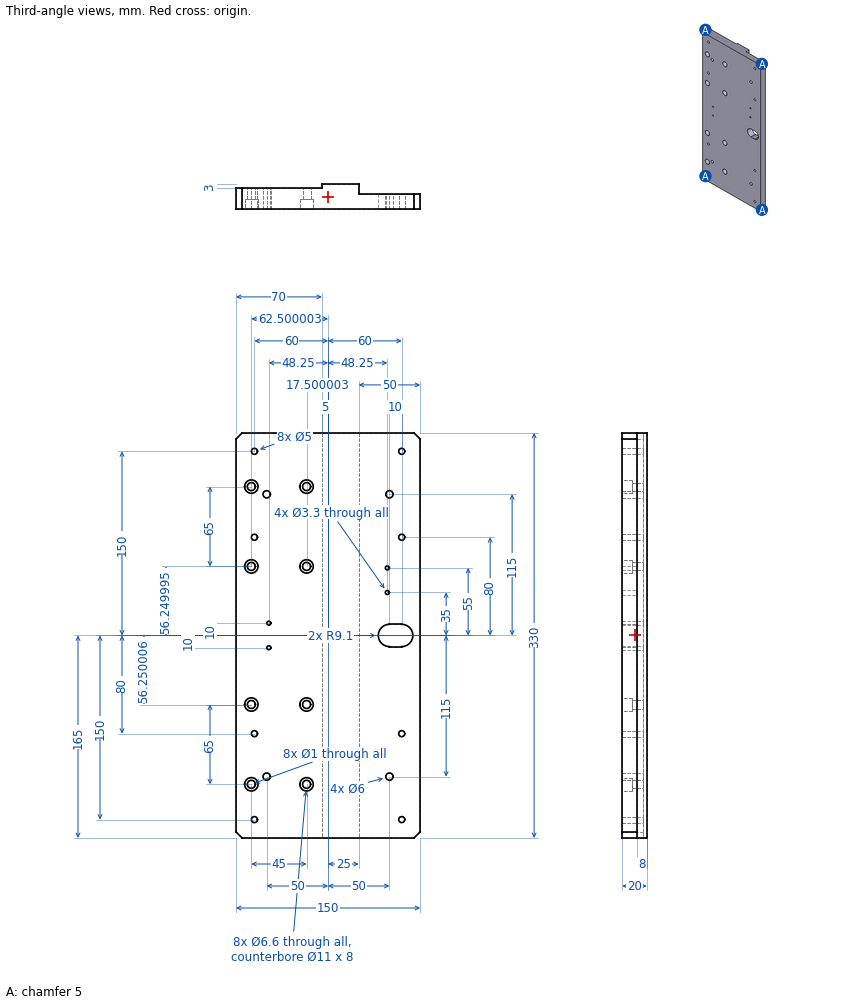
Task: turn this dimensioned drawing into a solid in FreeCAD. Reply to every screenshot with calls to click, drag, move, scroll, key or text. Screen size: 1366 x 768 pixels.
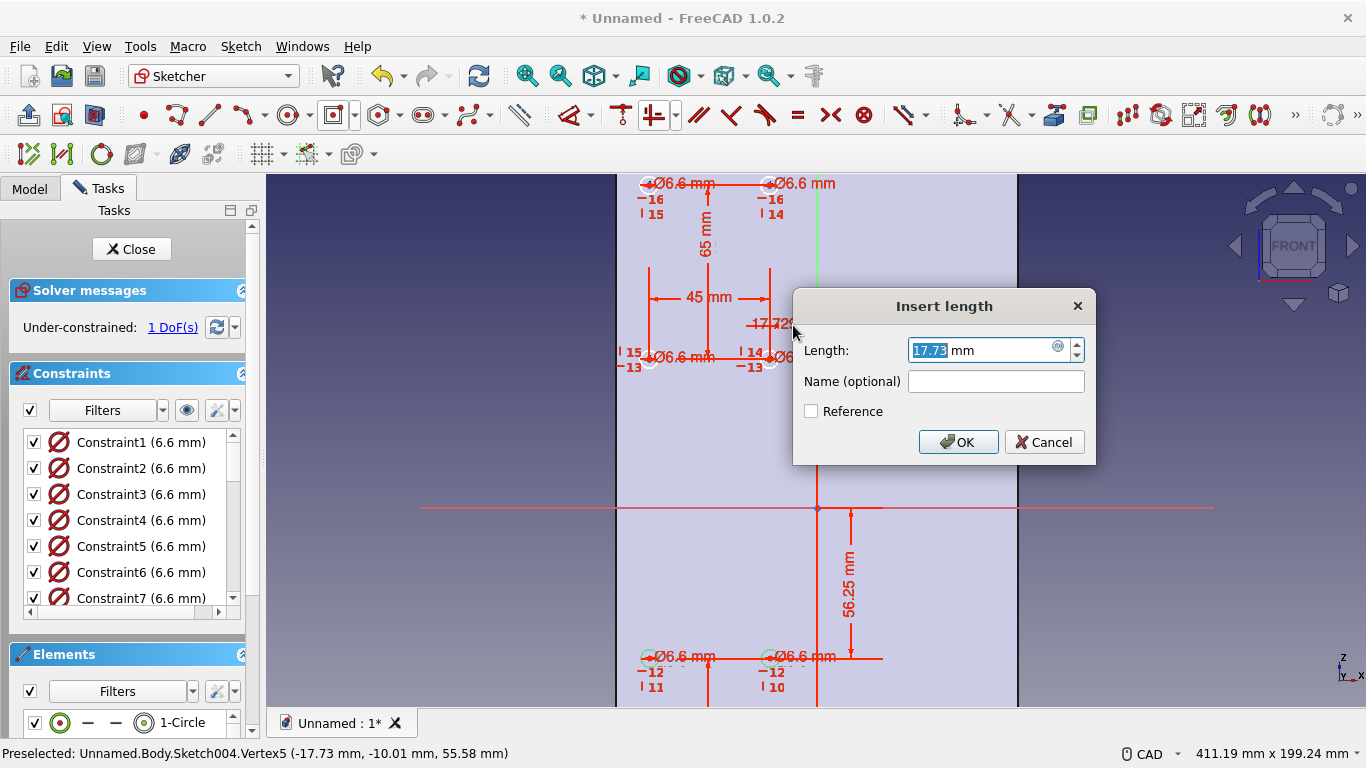
text(17.500003)
key(Return)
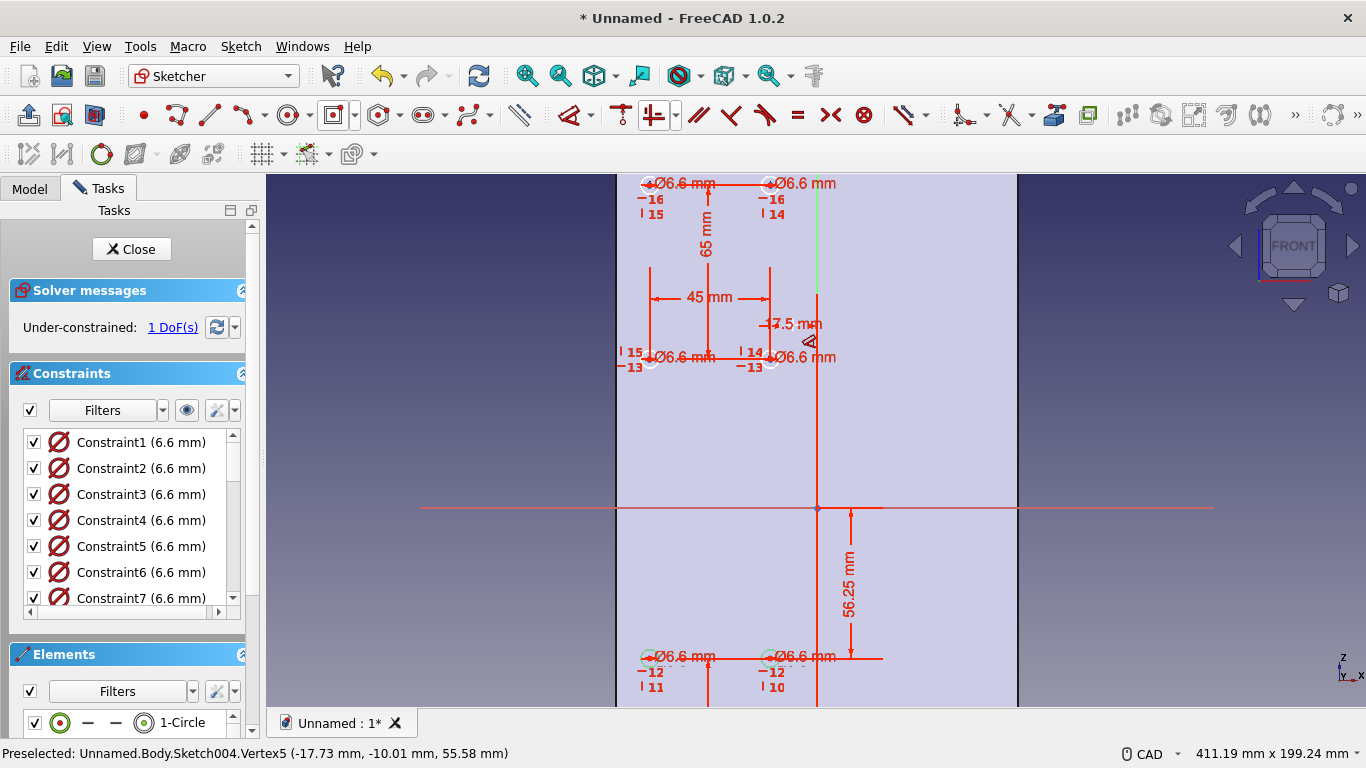
click(770, 359)
click(851, 434)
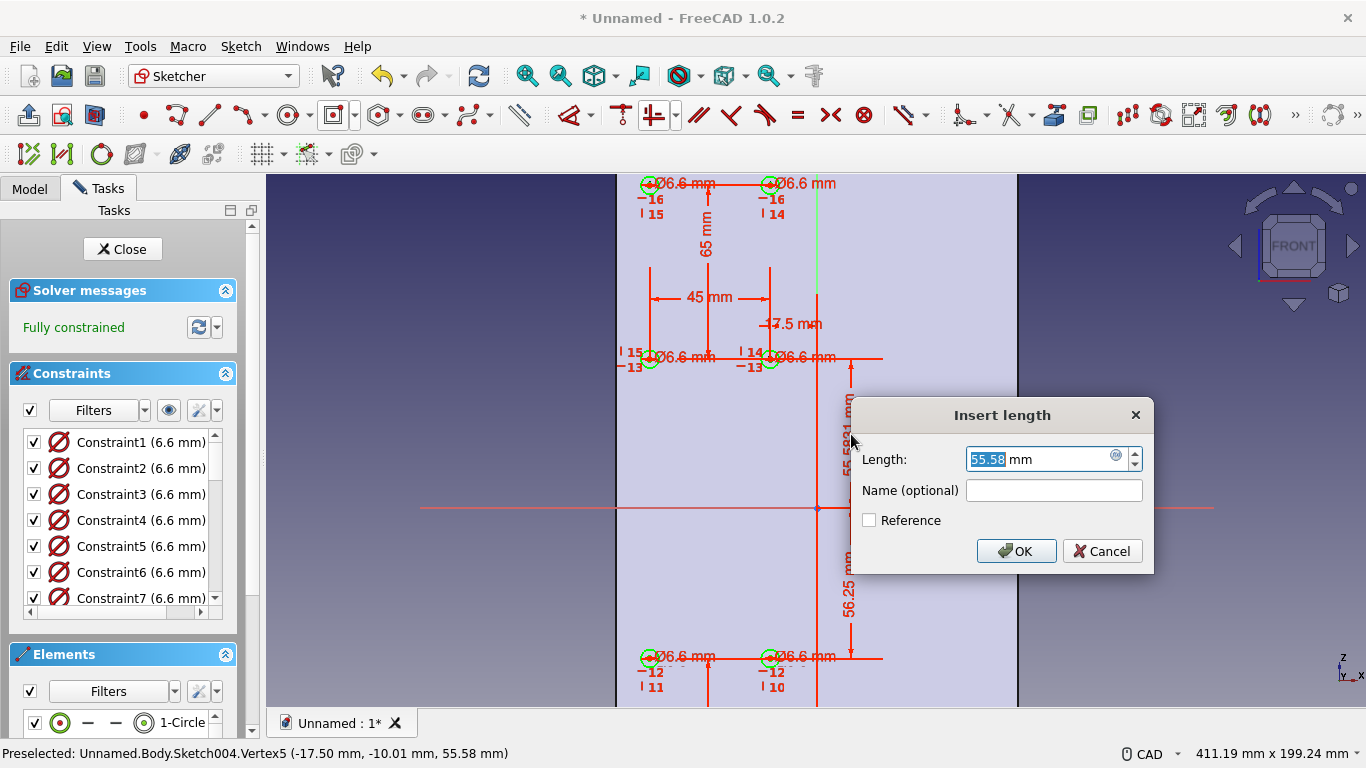
text(56.249995)
key(Return)
key(Escape)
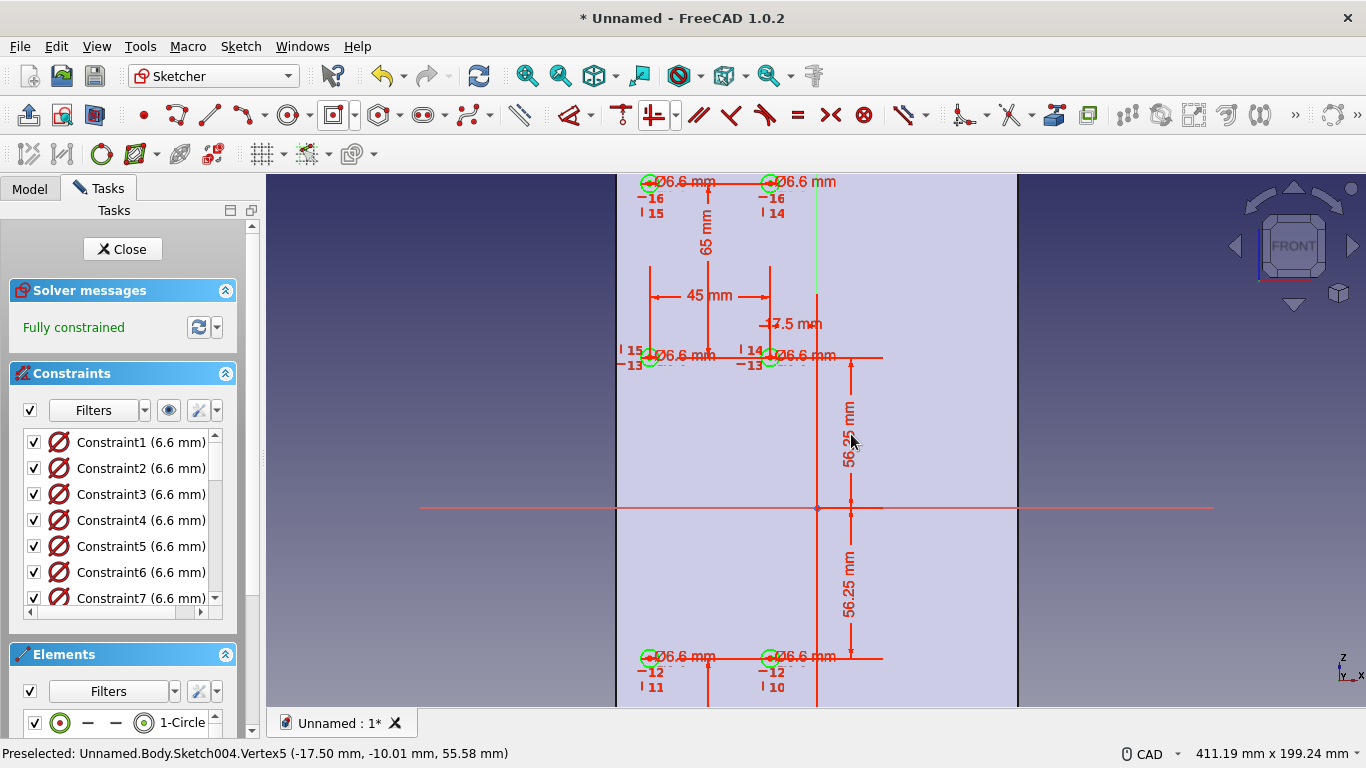
click(123, 249)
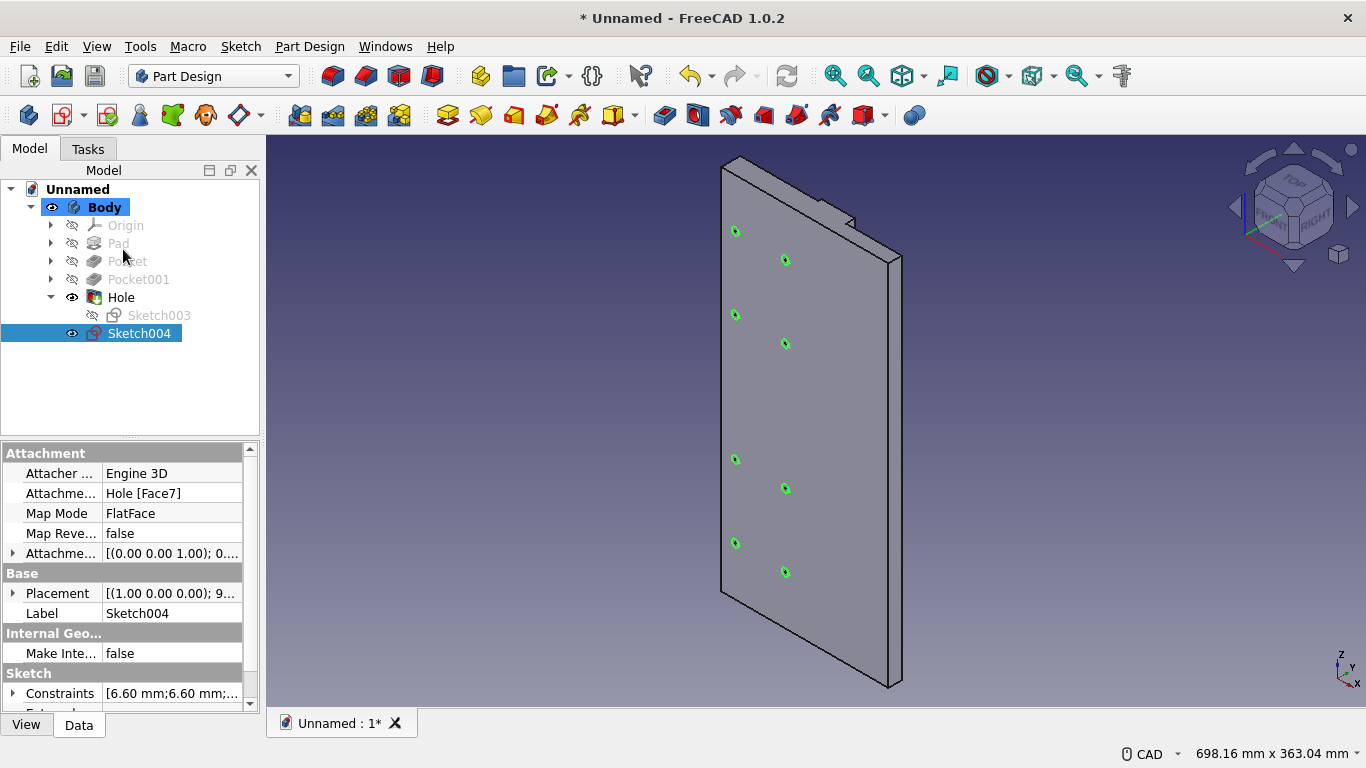
click(698, 116)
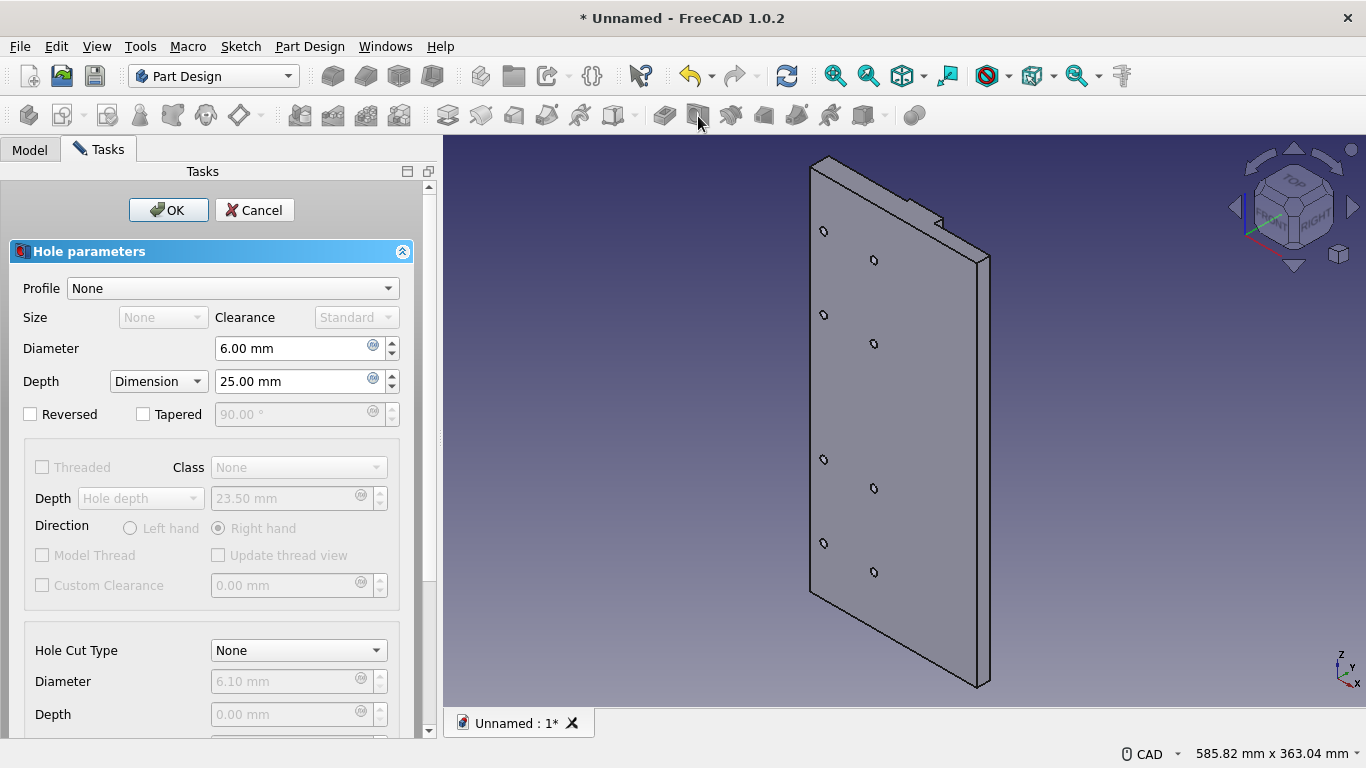
triple_click(300, 348)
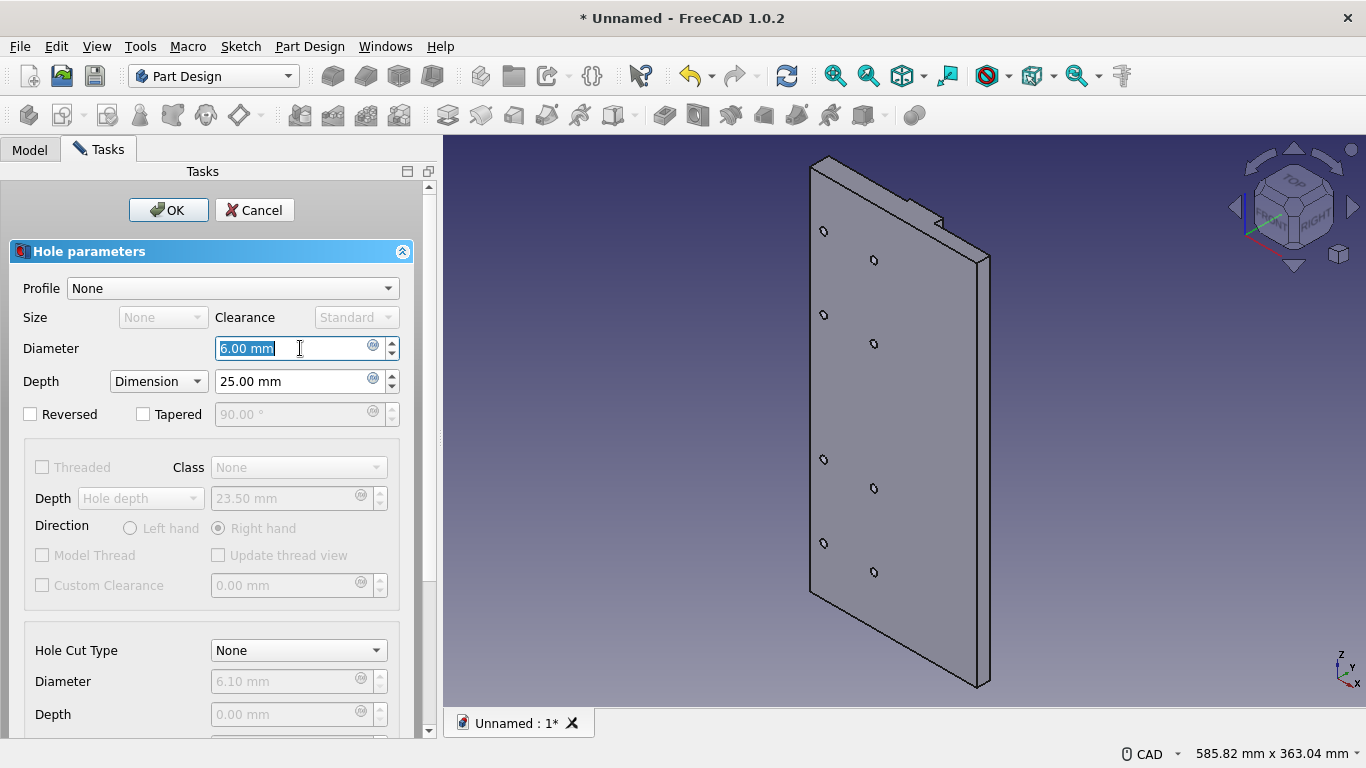
text(6.6)
key(Tab)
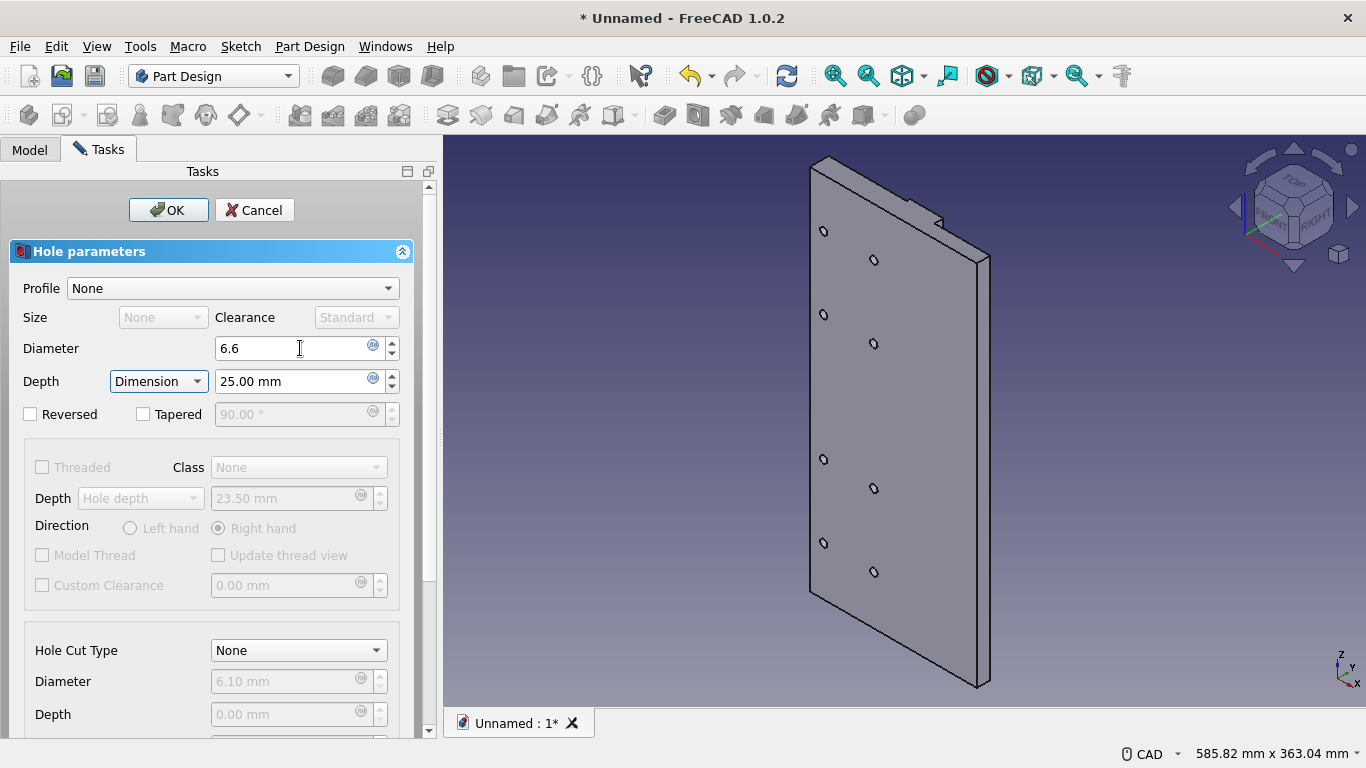
click(160, 382)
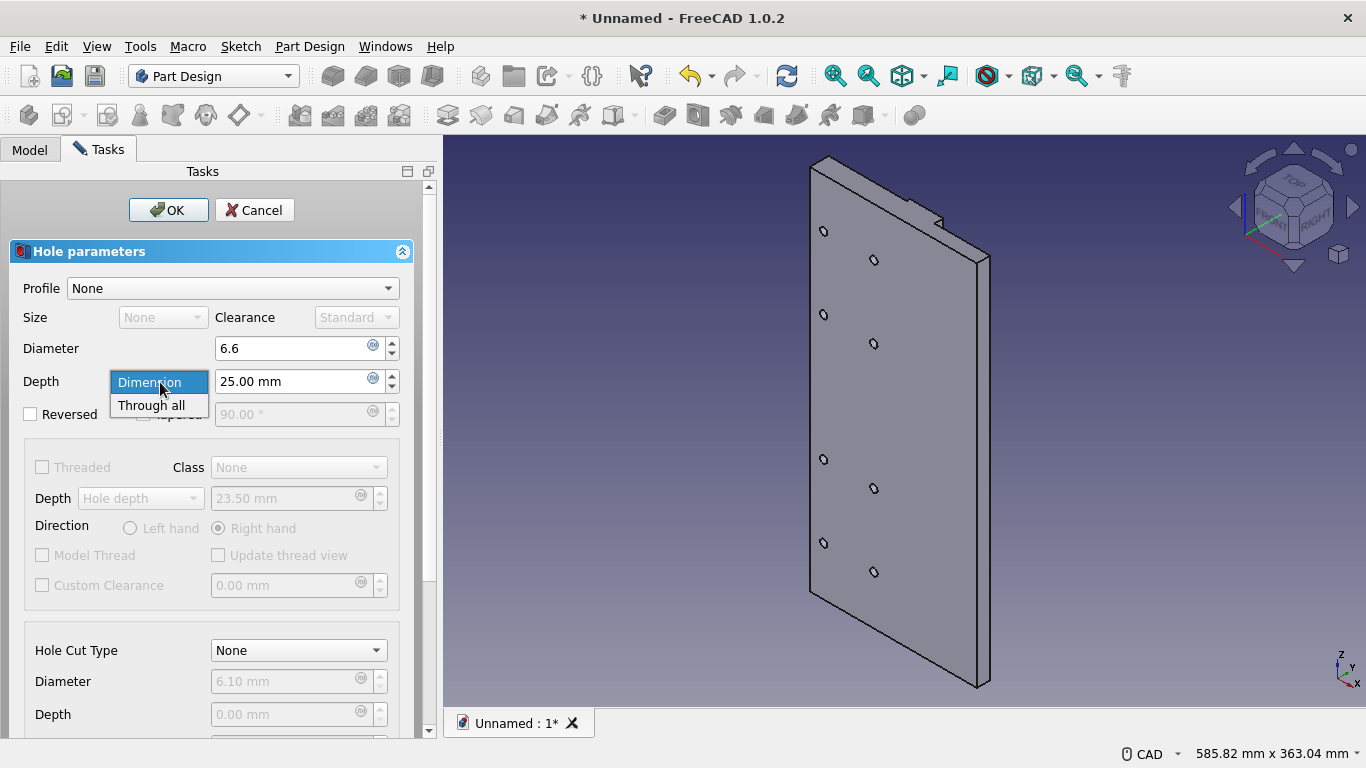
click(158, 406)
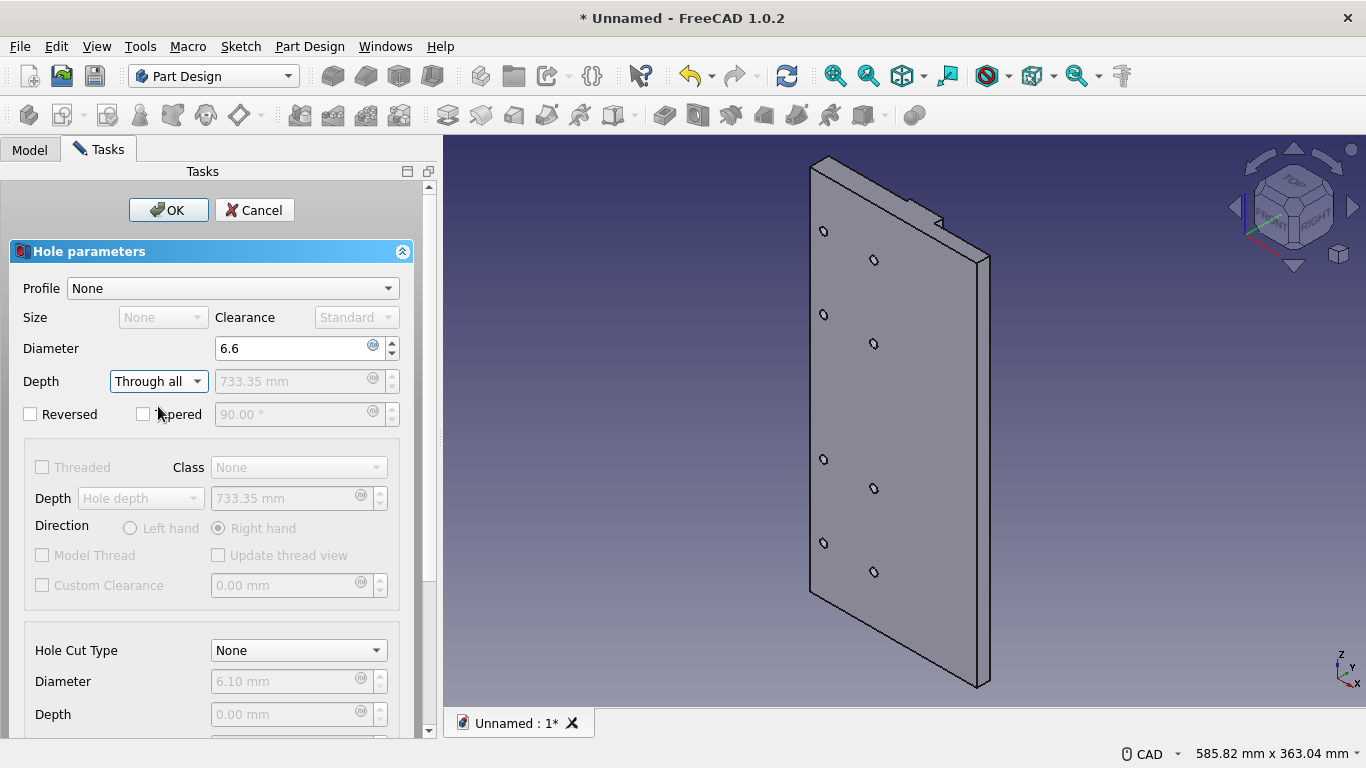
click(300, 650)